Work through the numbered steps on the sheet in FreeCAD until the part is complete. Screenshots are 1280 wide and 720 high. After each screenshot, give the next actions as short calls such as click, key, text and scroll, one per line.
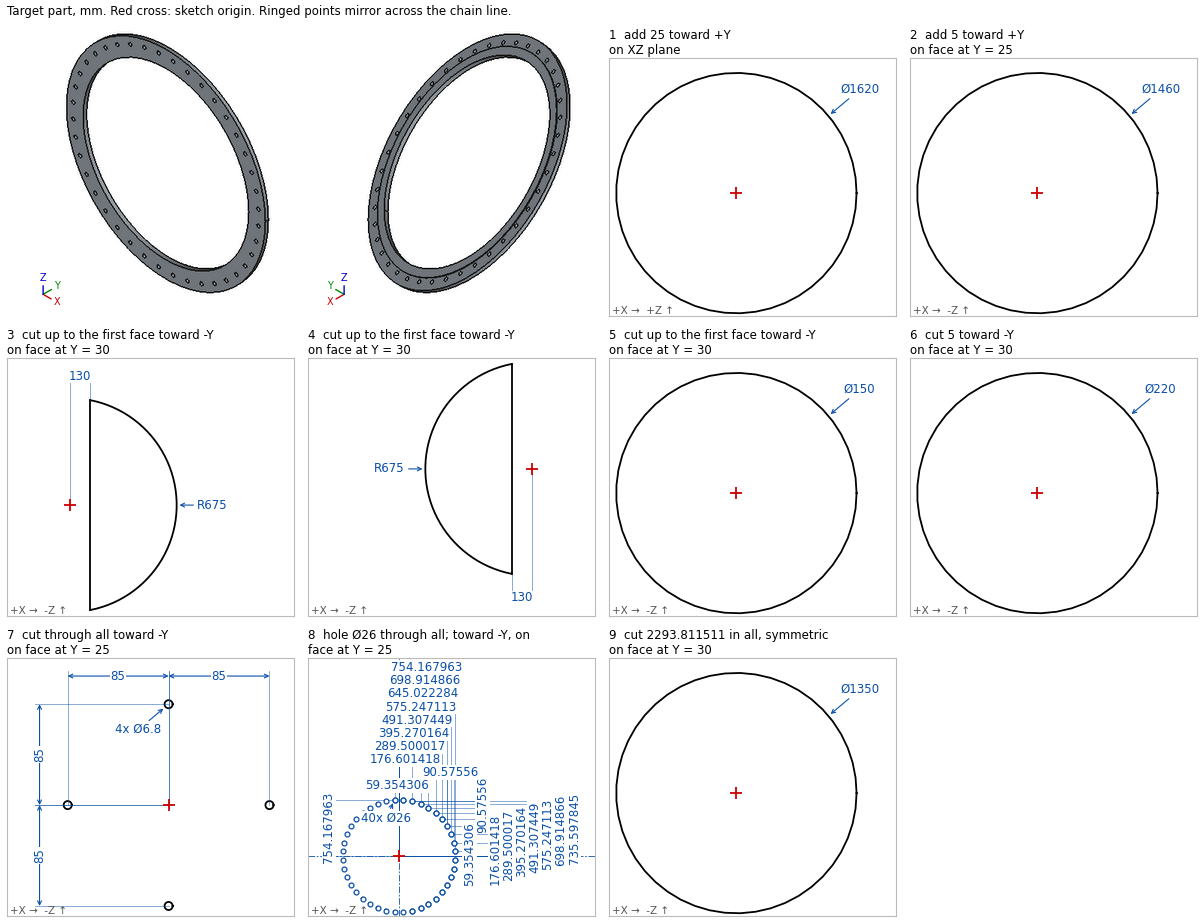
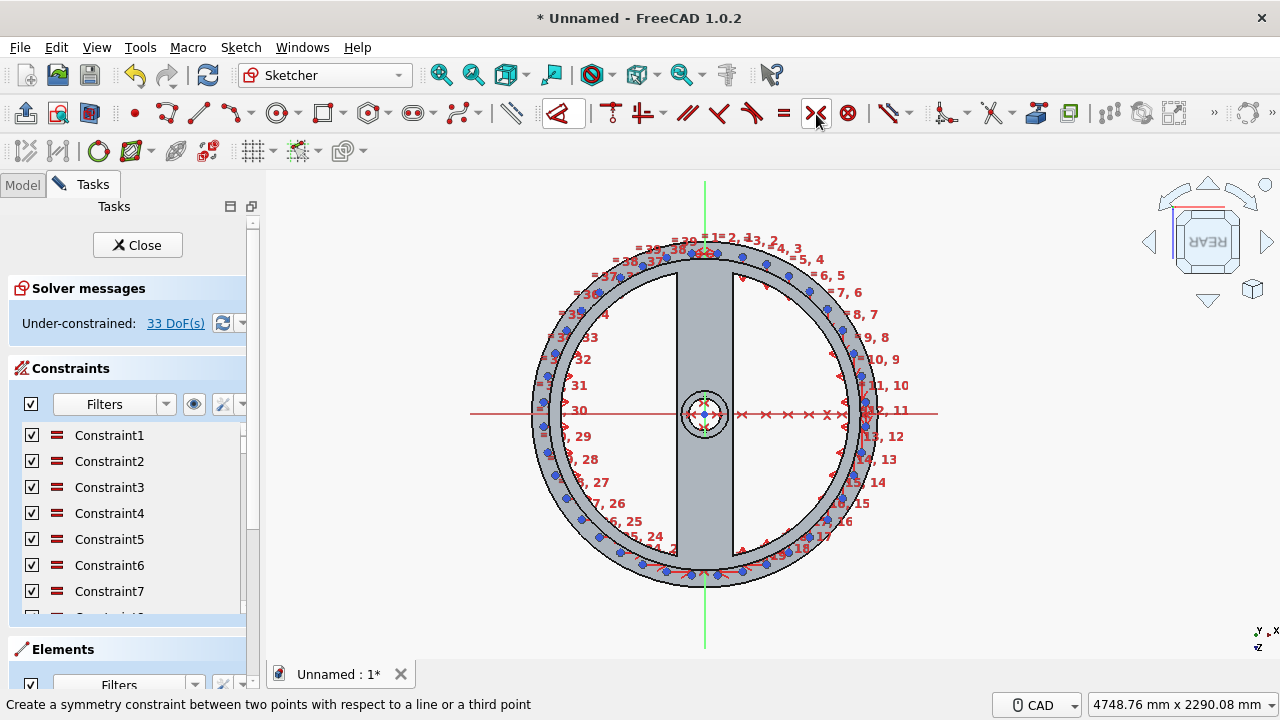
click(843, 330)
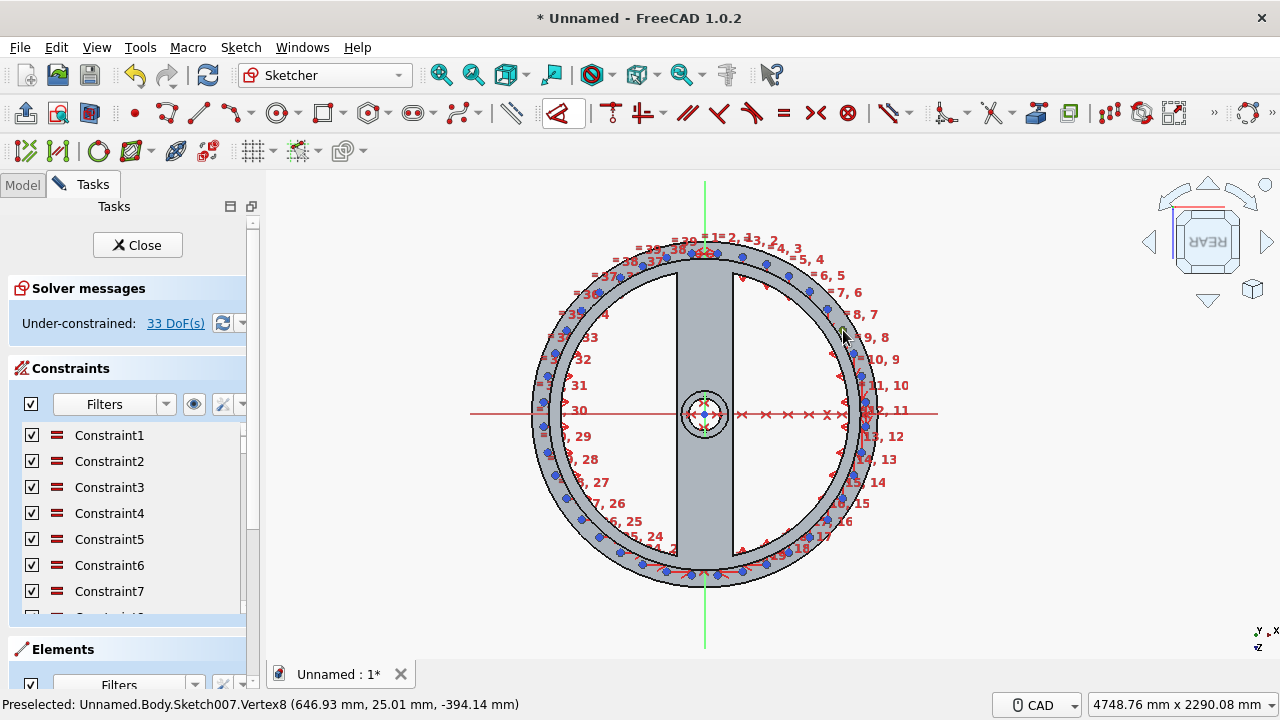
click(567, 331)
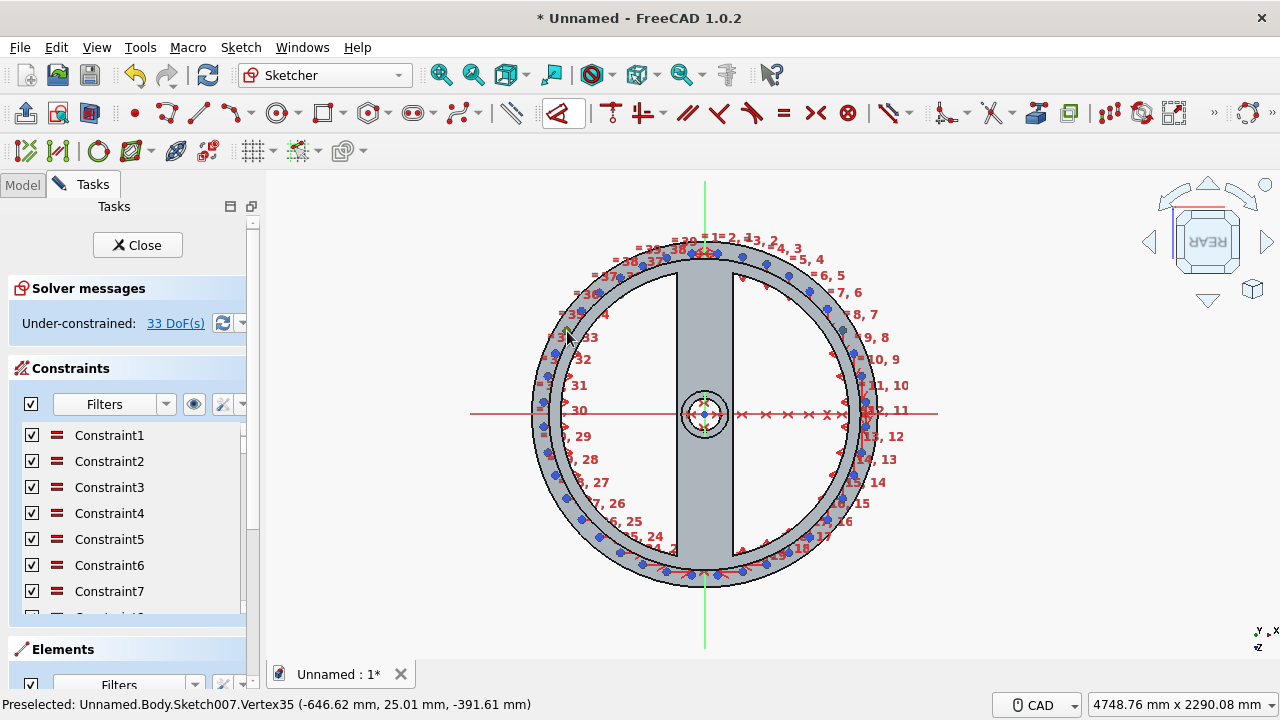
click(705, 507)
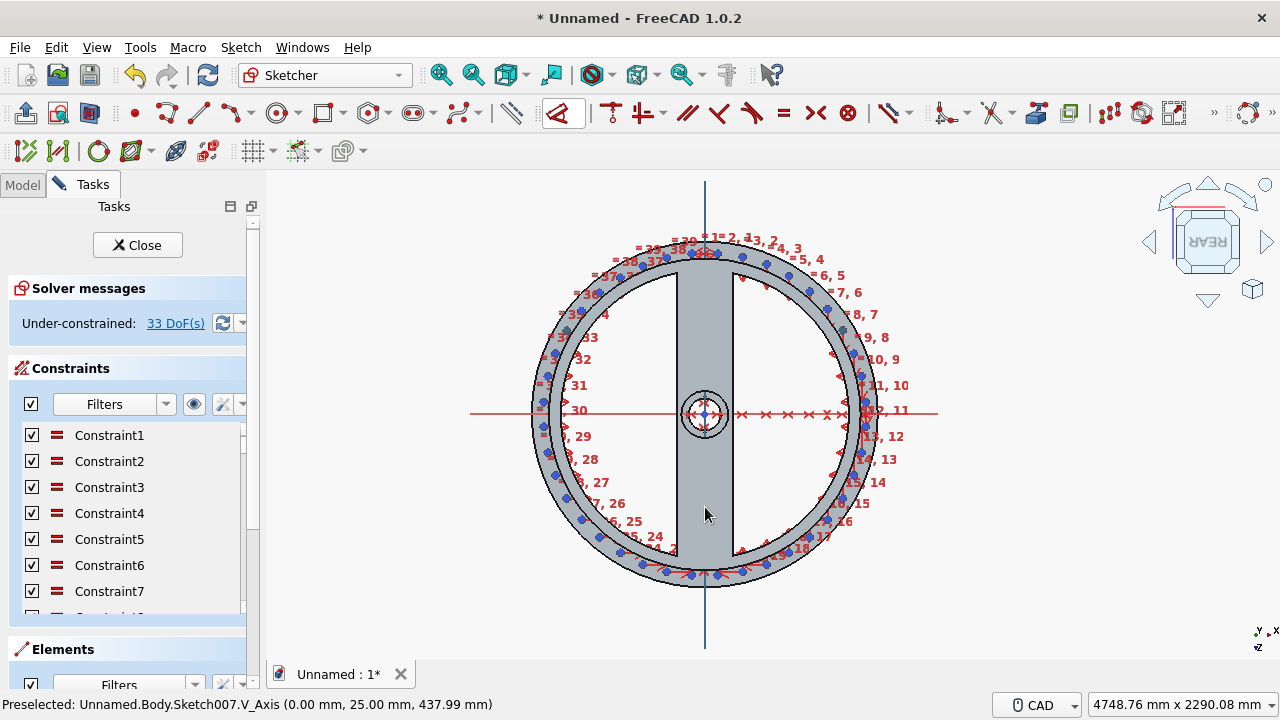
key(s)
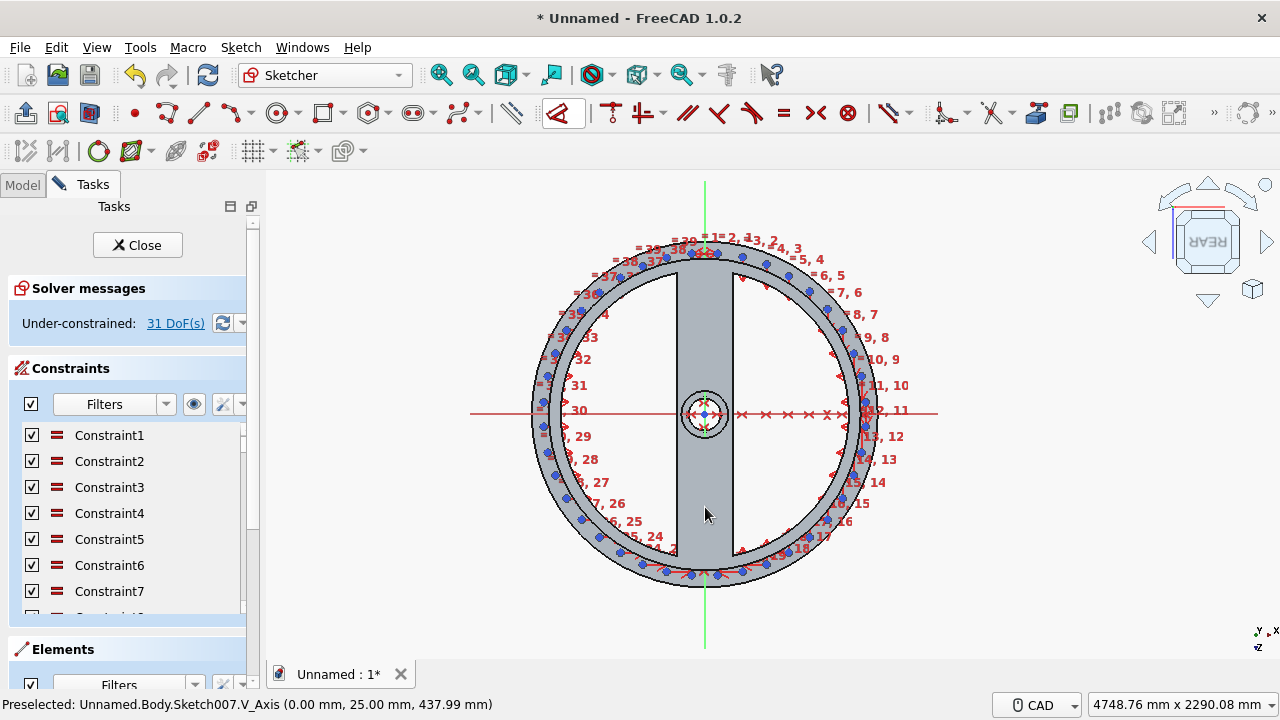
click(828, 309)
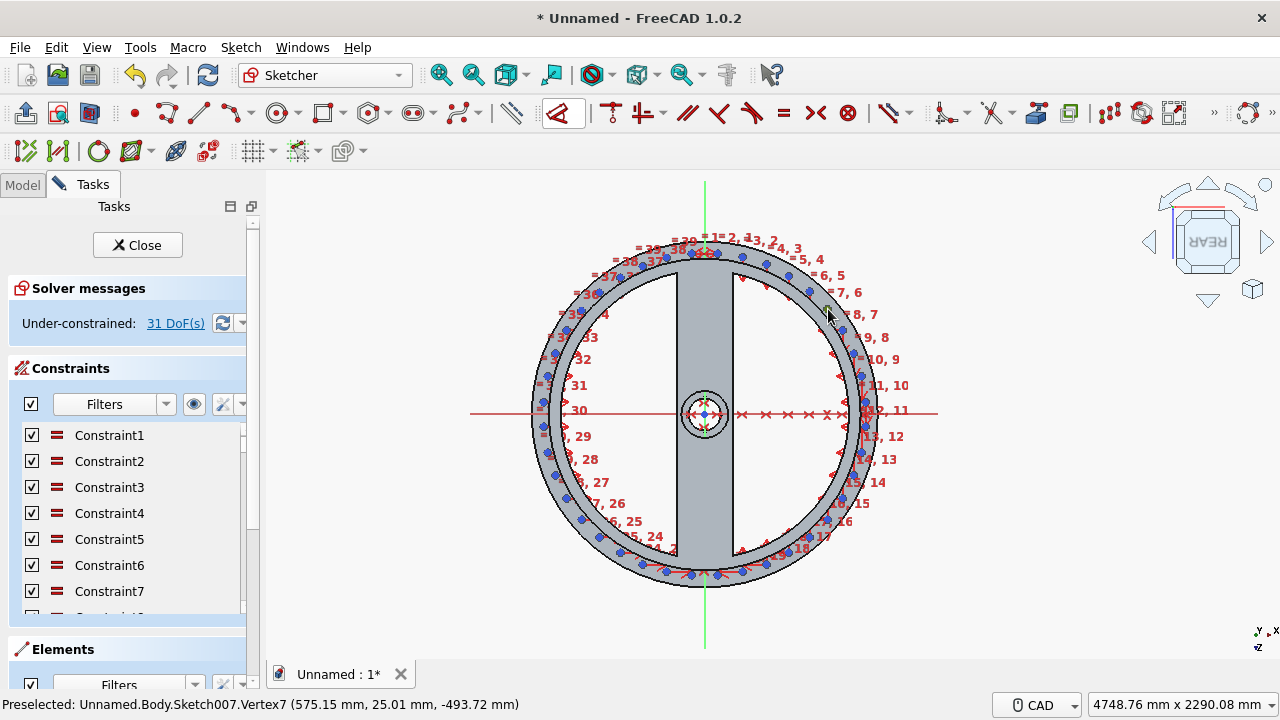
click(582, 311)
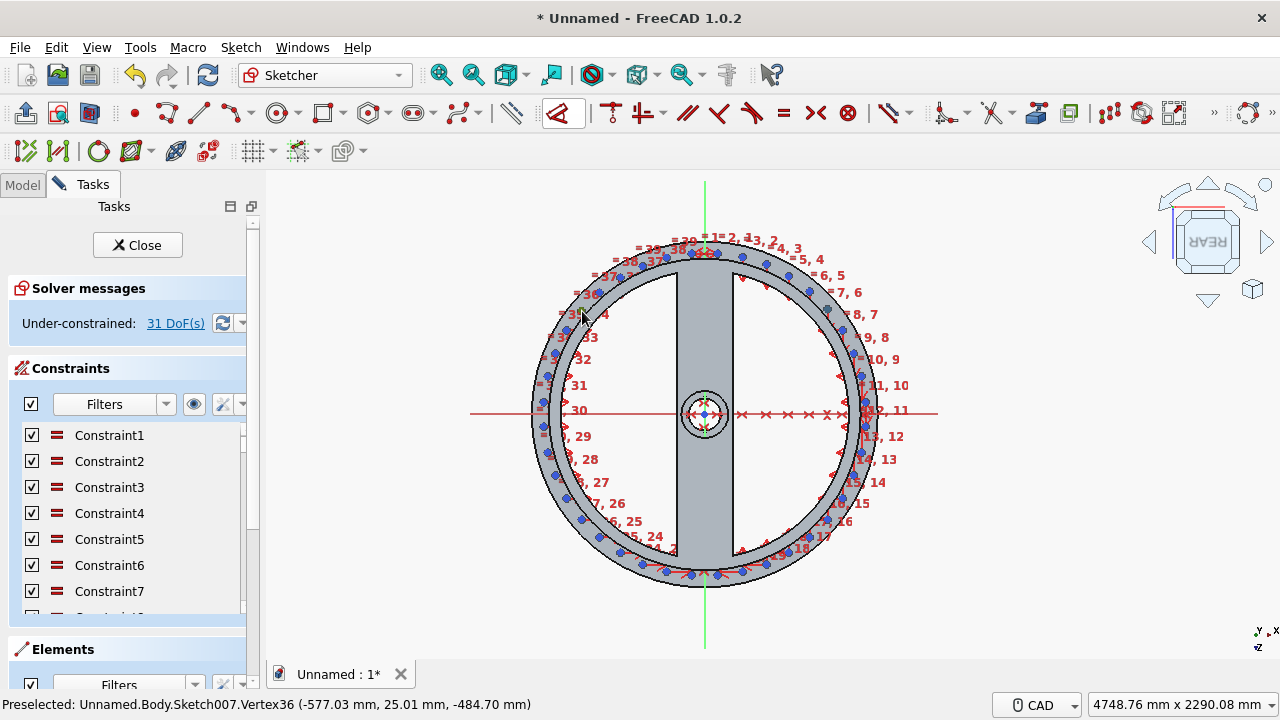
click(705, 507)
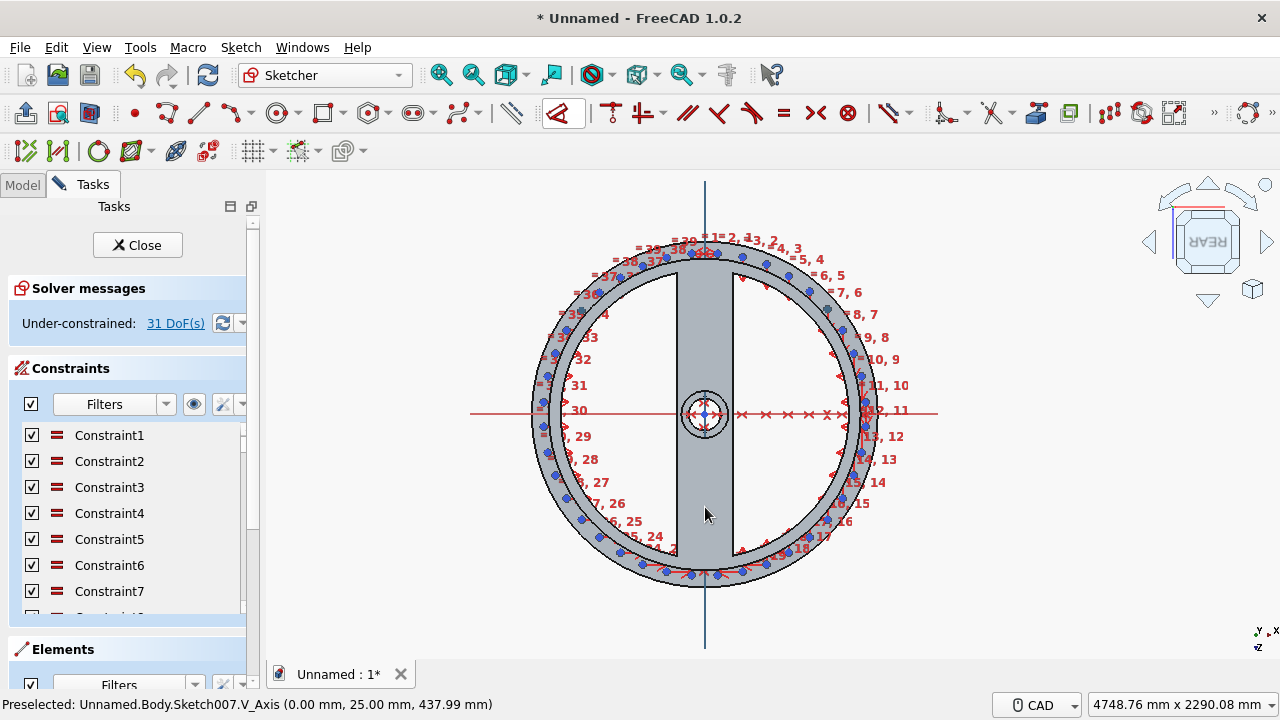
click(816, 114)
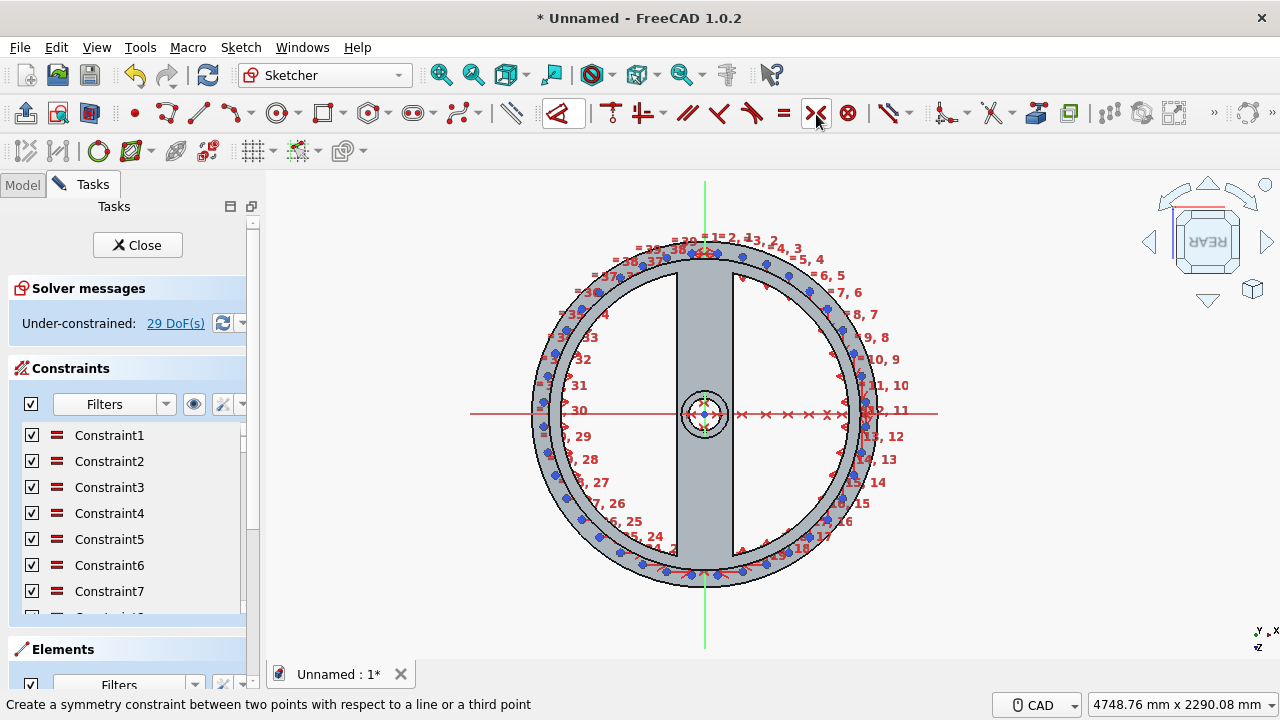
click(810, 292)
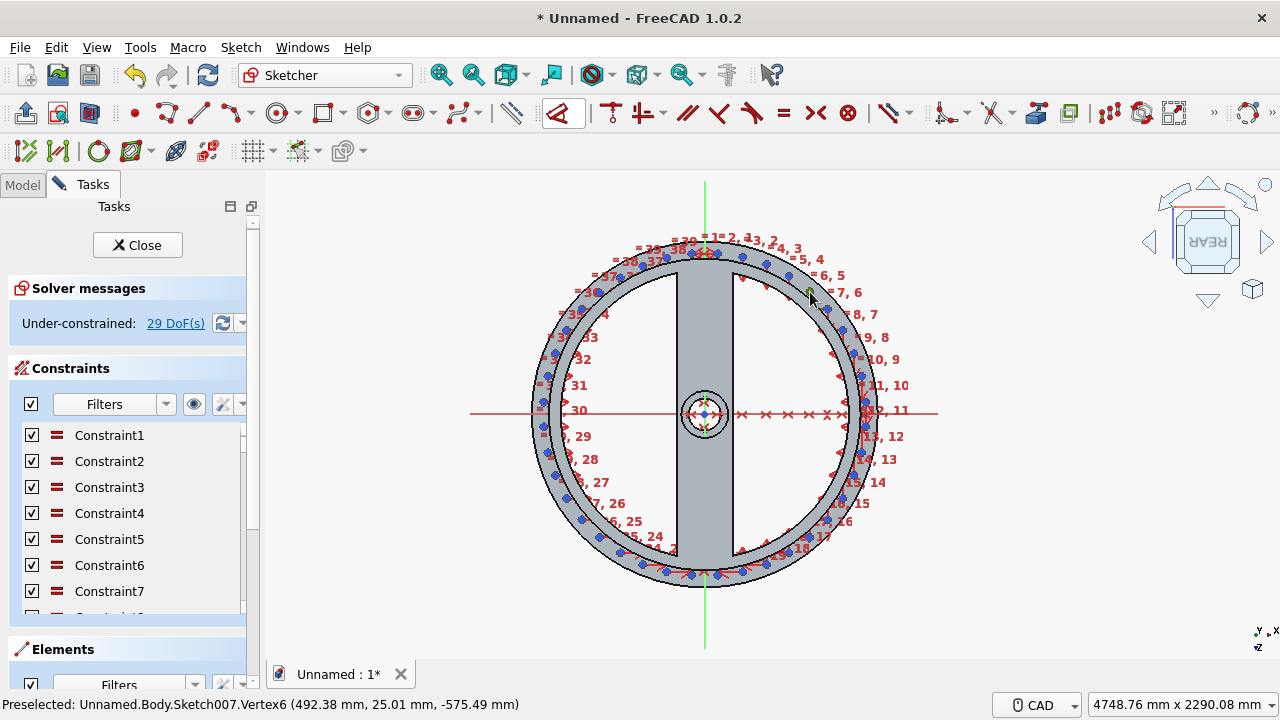
click(599, 293)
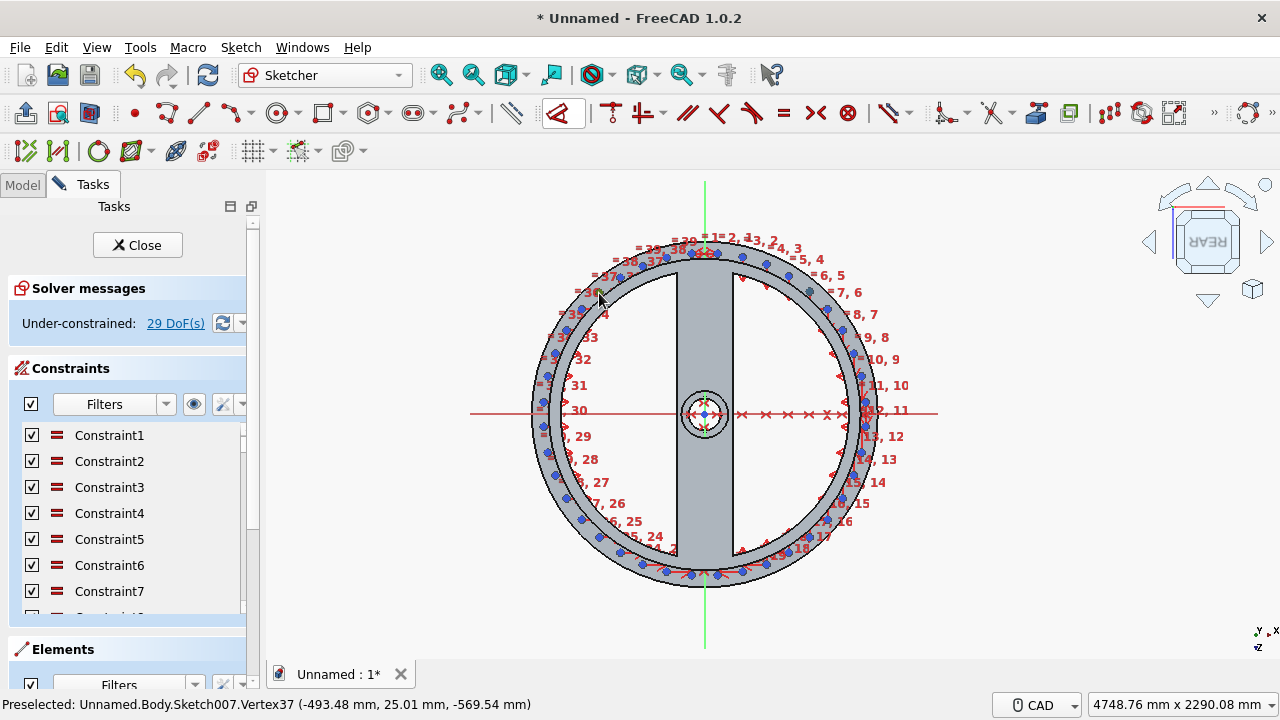
click(705, 507)